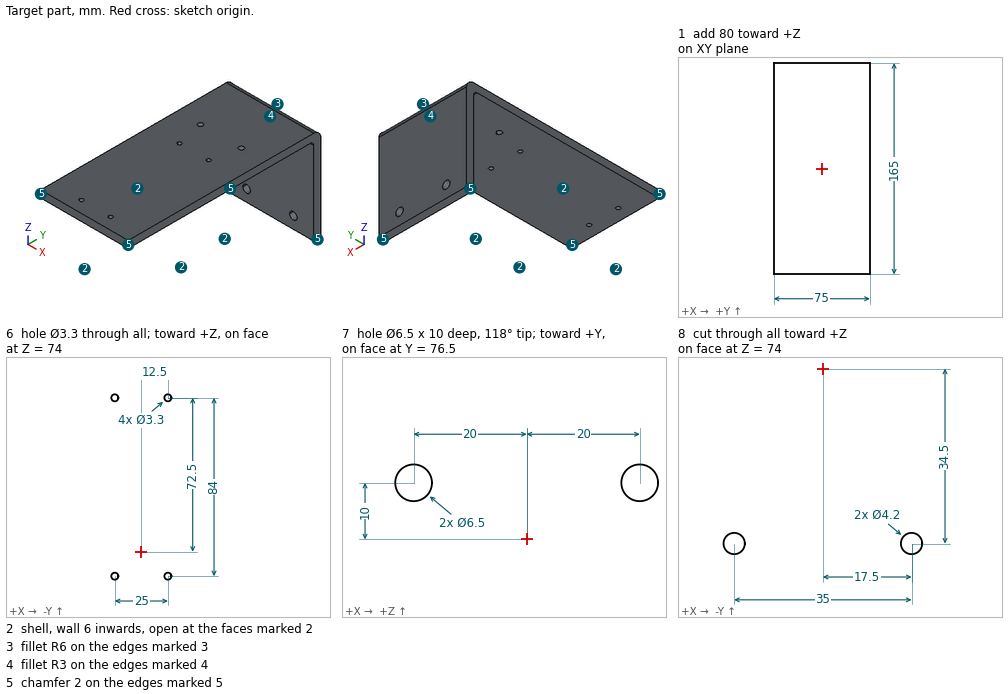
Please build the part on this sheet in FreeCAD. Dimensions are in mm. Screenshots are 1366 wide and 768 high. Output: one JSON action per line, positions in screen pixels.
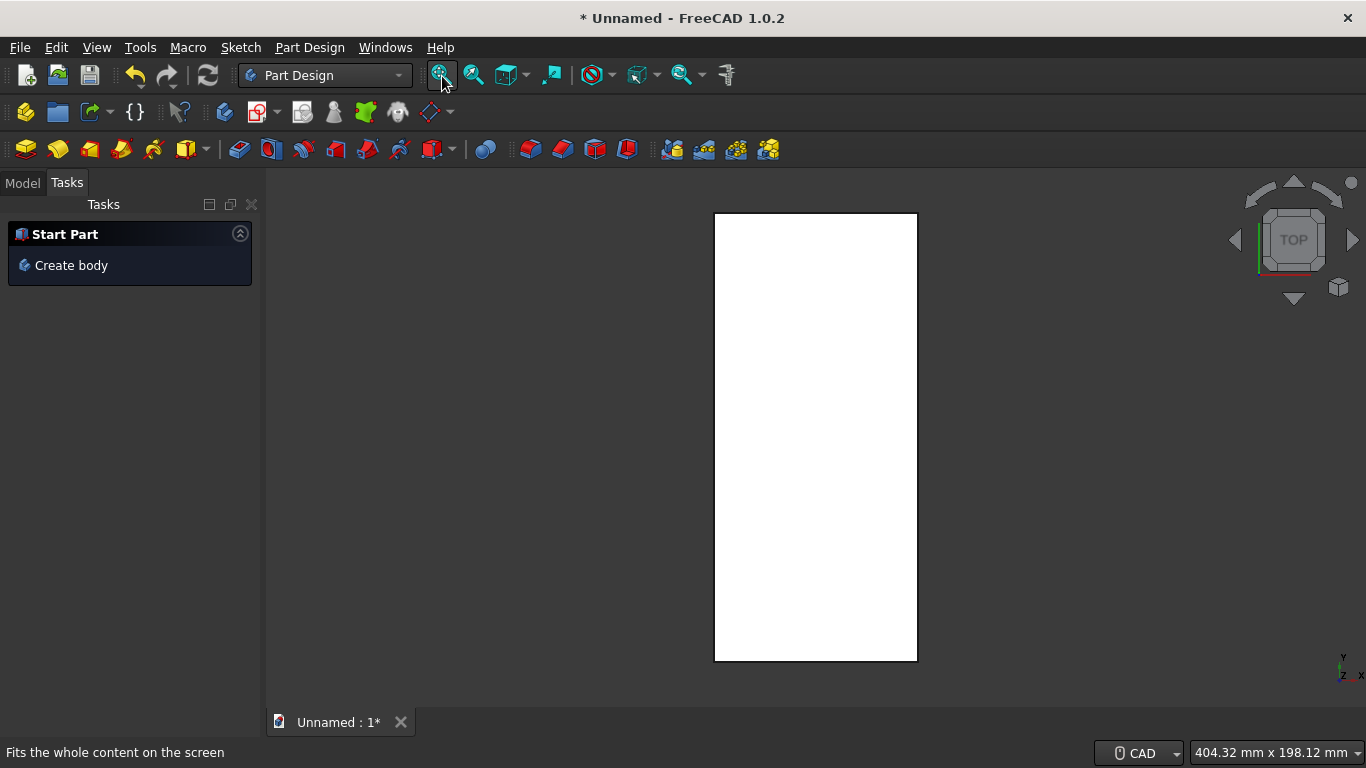
{"action": "left_click", "coordinate": [816, 212]}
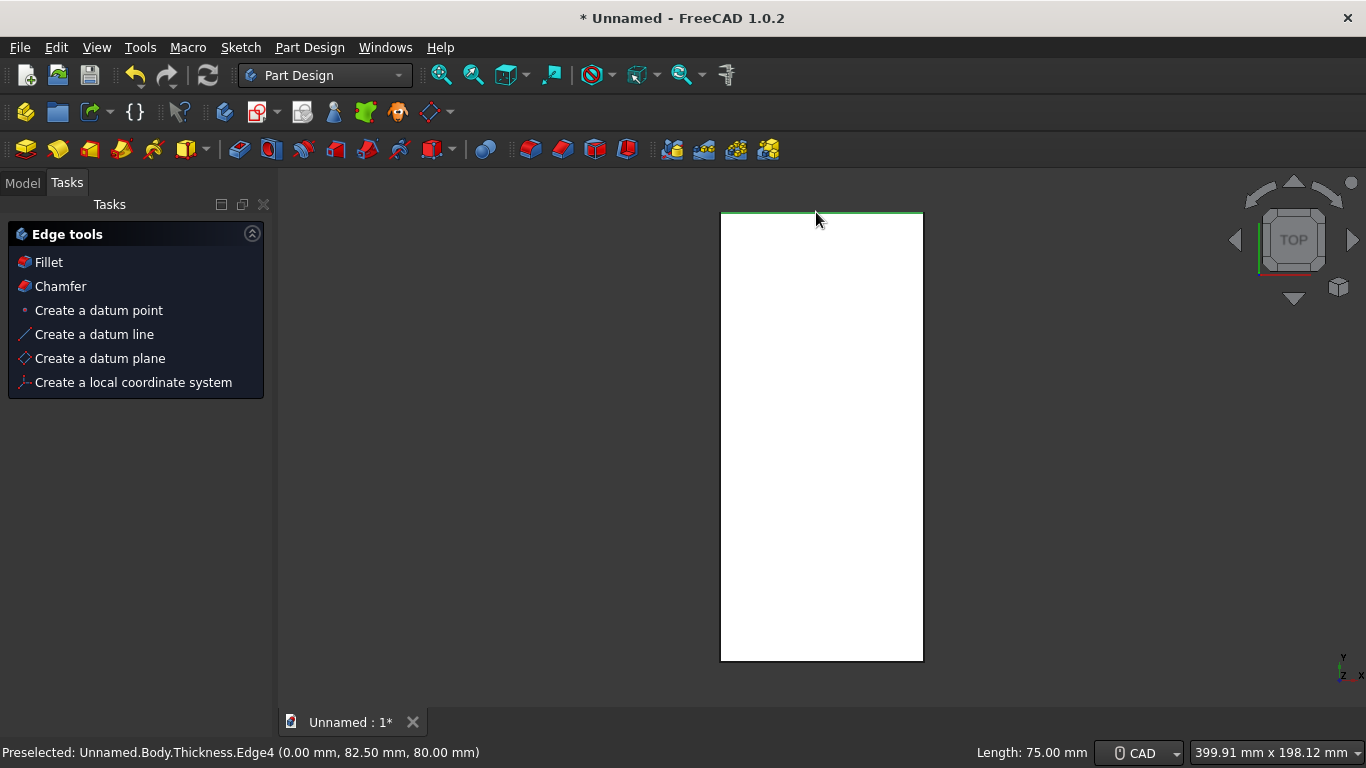
{"action": "left_click", "coordinate": [532, 150]}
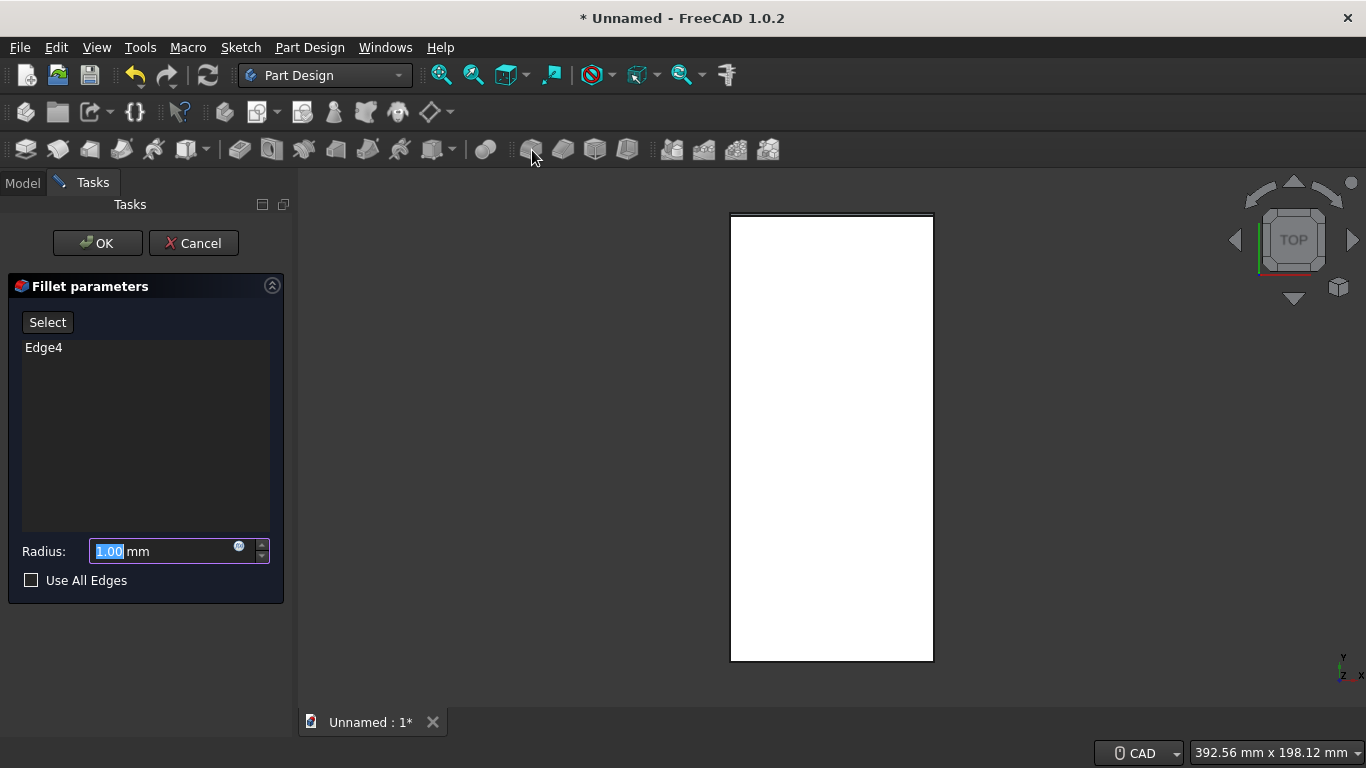
{"action": "type", "text": "6"}
{"action": "key", "text": "Tab"}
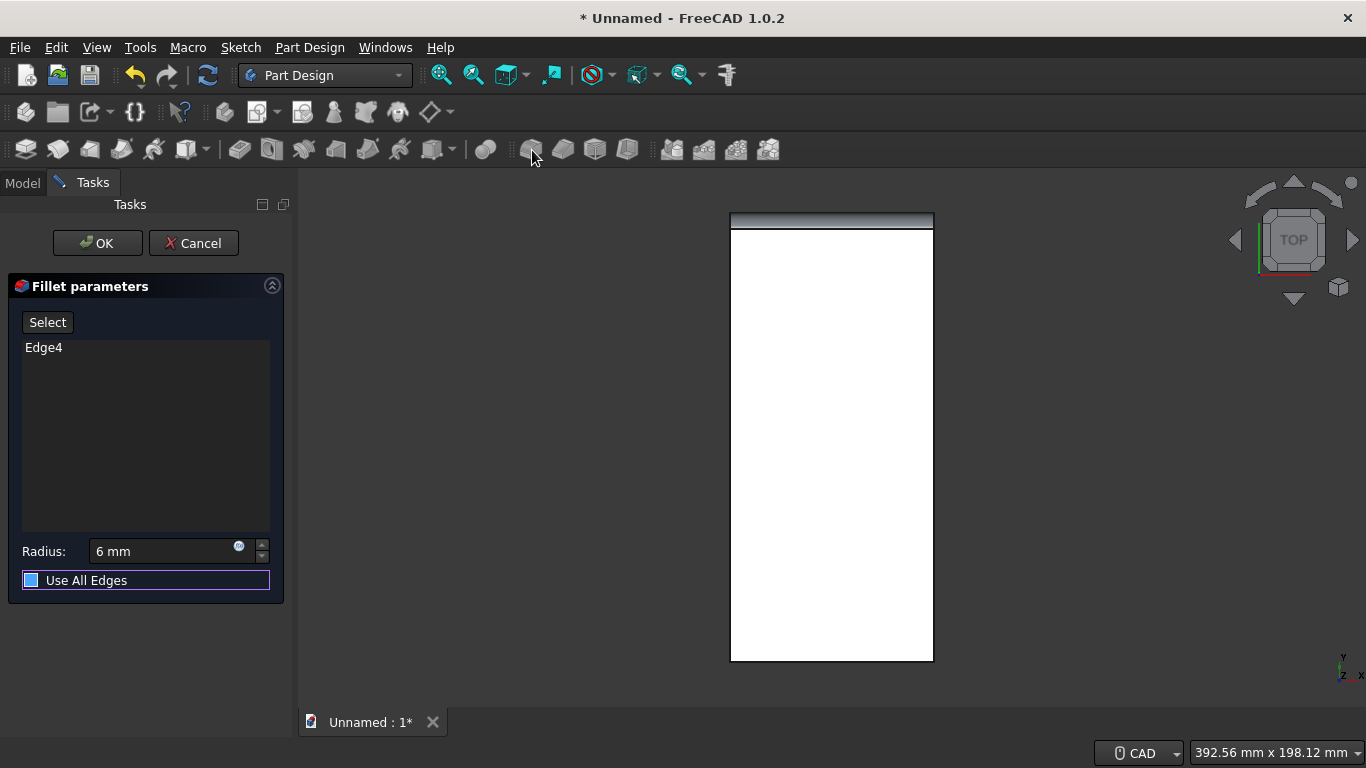
{"action": "left_click", "coordinate": [98, 243]}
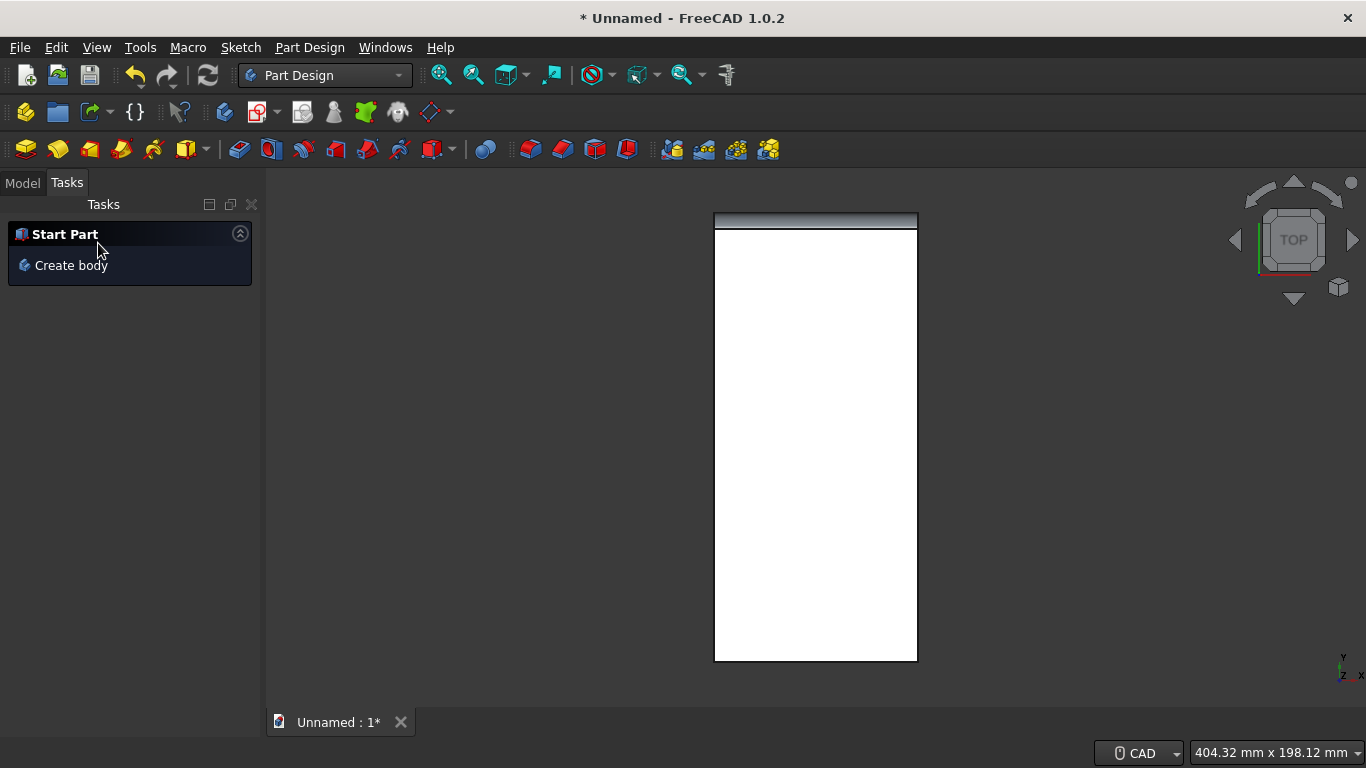
{"action": "key", "text": "0"}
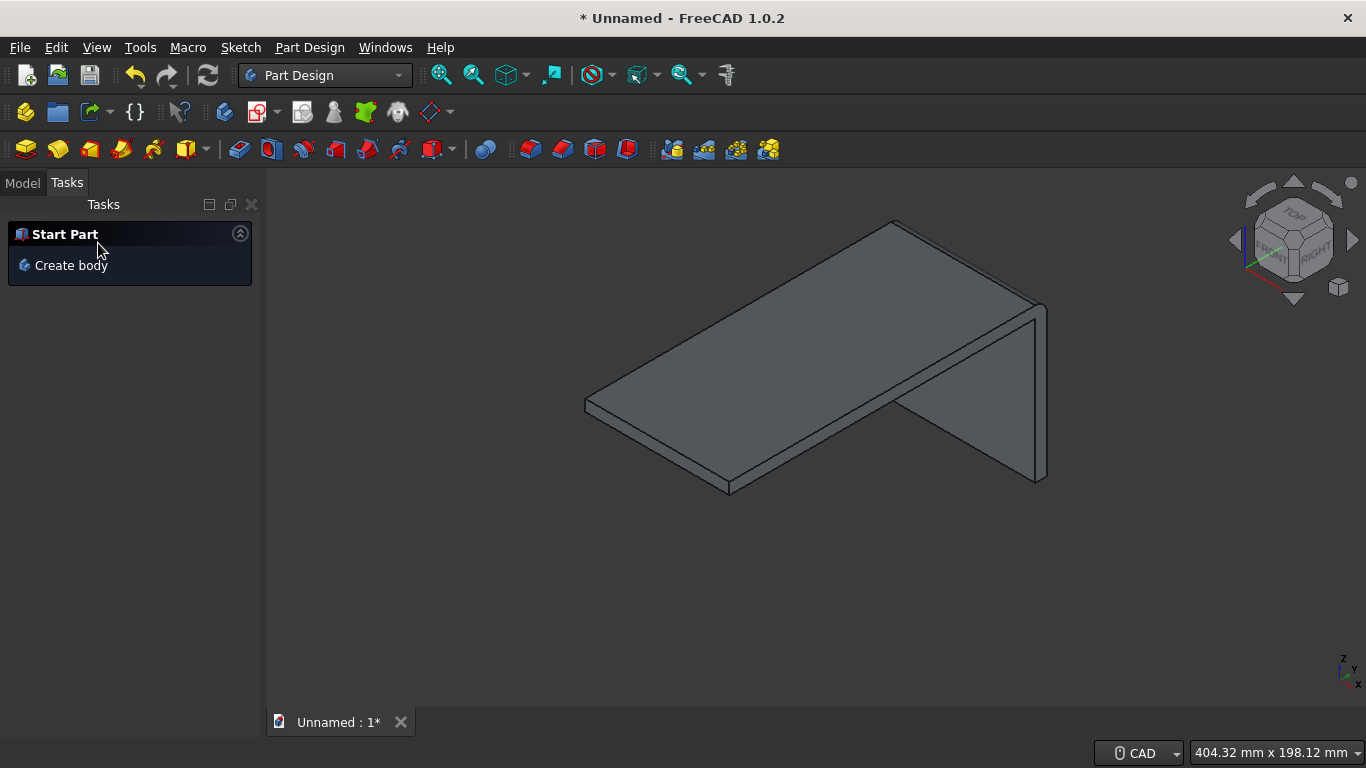
{"action": "key", "text": "2"}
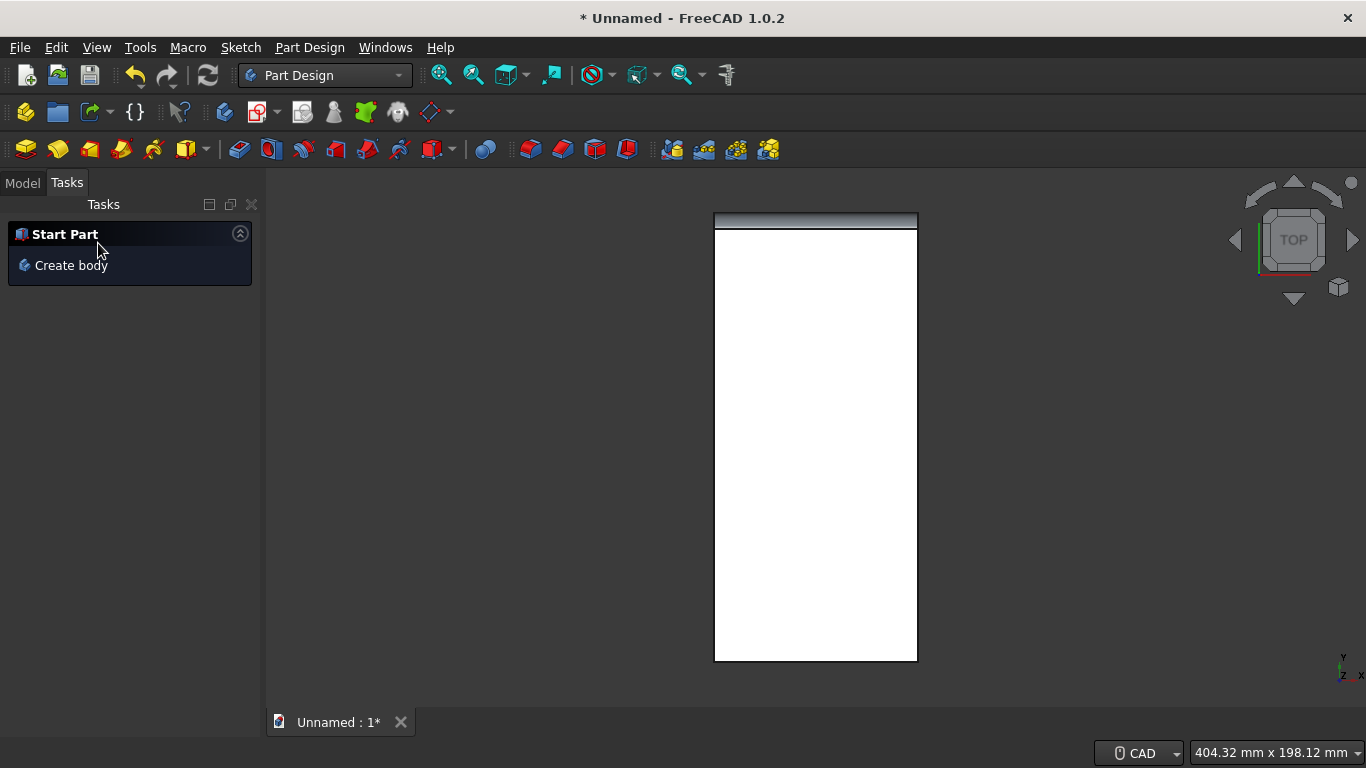
{"action": "key", "text": "1"}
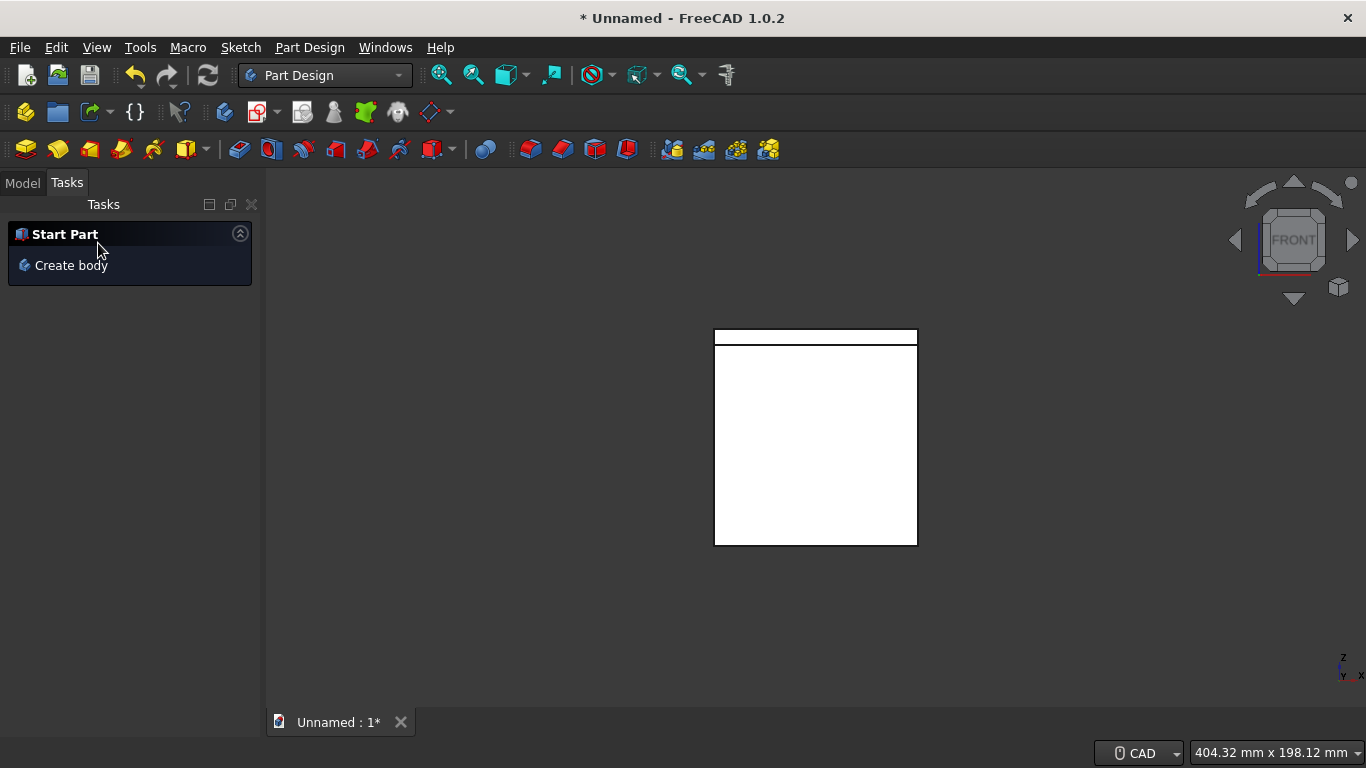
{"action": "left_click", "coordinate": [442, 76]}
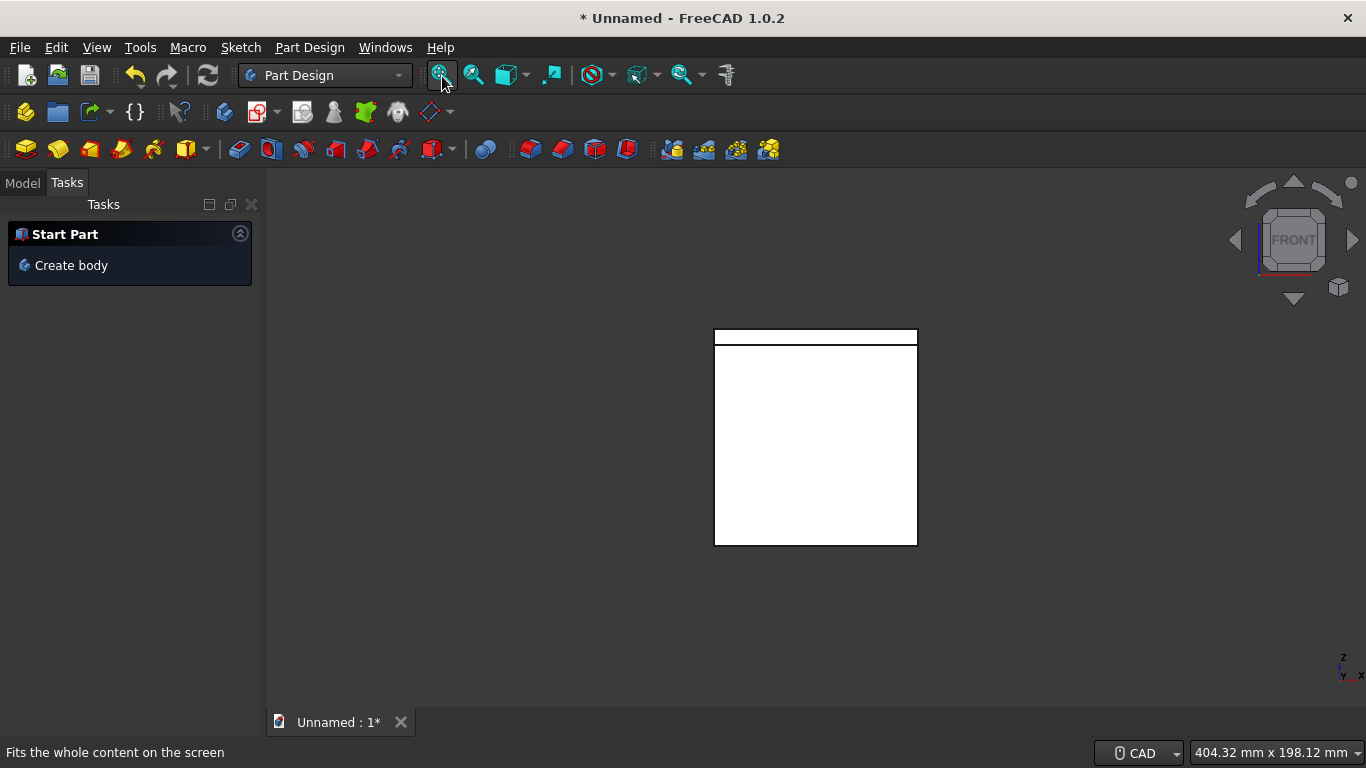
{"action": "key", "text": "3"}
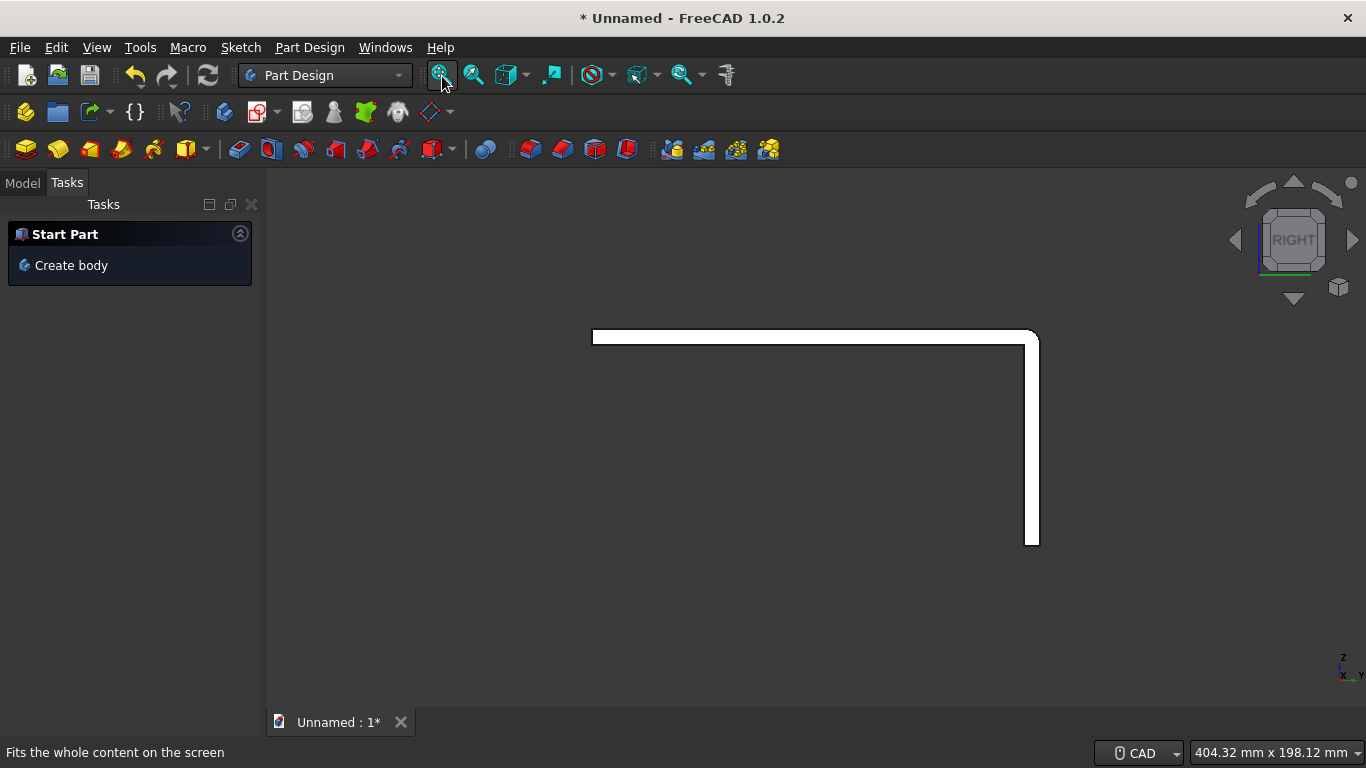
{"action": "left_click", "coordinate": [442, 76]}